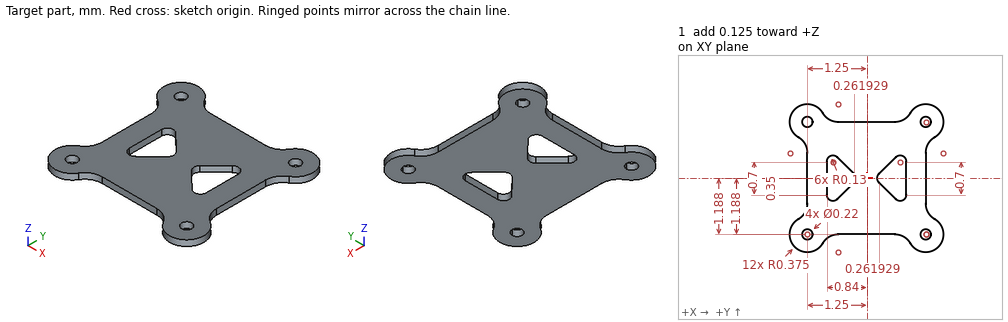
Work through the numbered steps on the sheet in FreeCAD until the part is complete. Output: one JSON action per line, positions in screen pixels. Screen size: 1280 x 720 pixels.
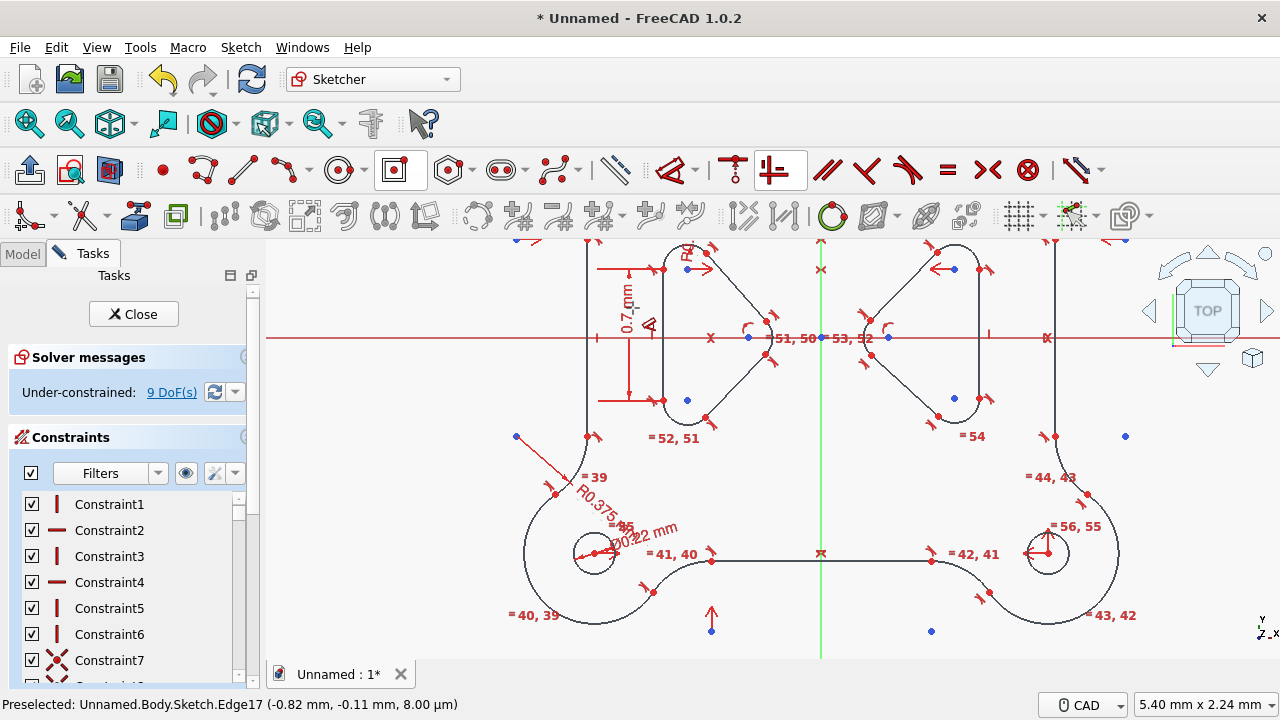
{"action": "left_click", "coordinate": [979, 308]}
{"action": "left_click", "coordinate": [1013, 304]}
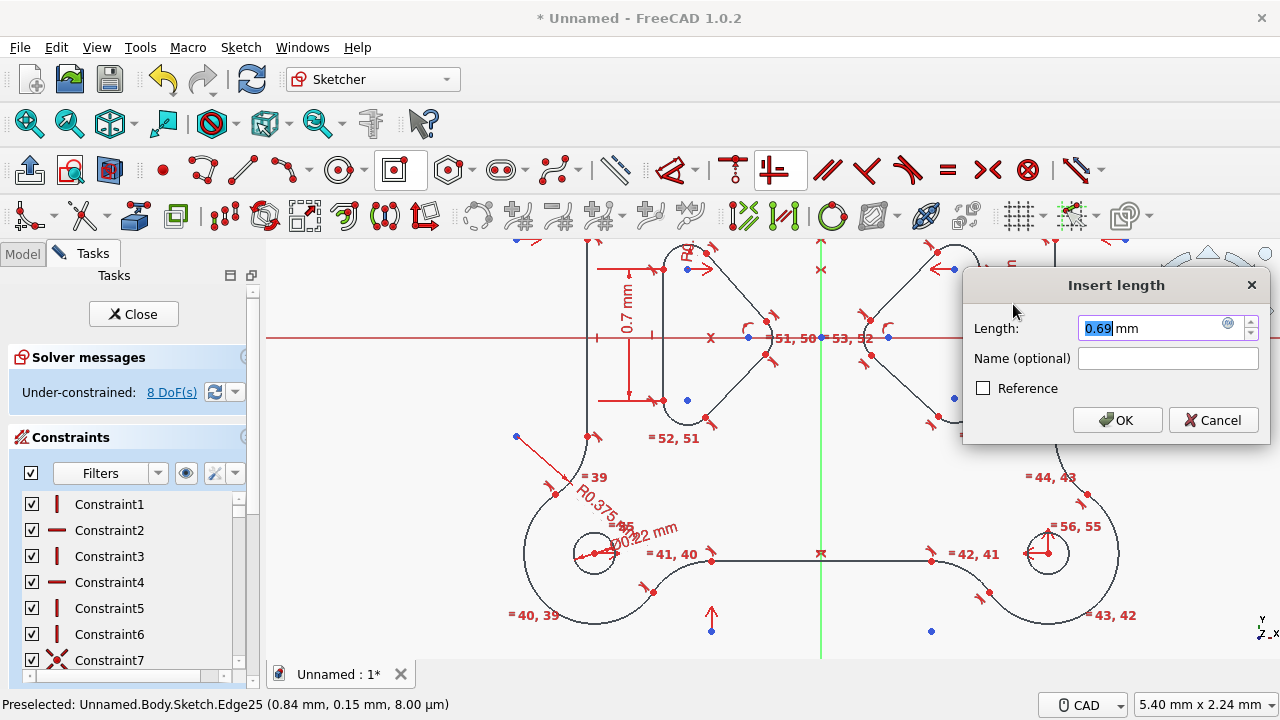
{"action": "type", "text": "0.7"}
{"action": "key", "text": "Return"}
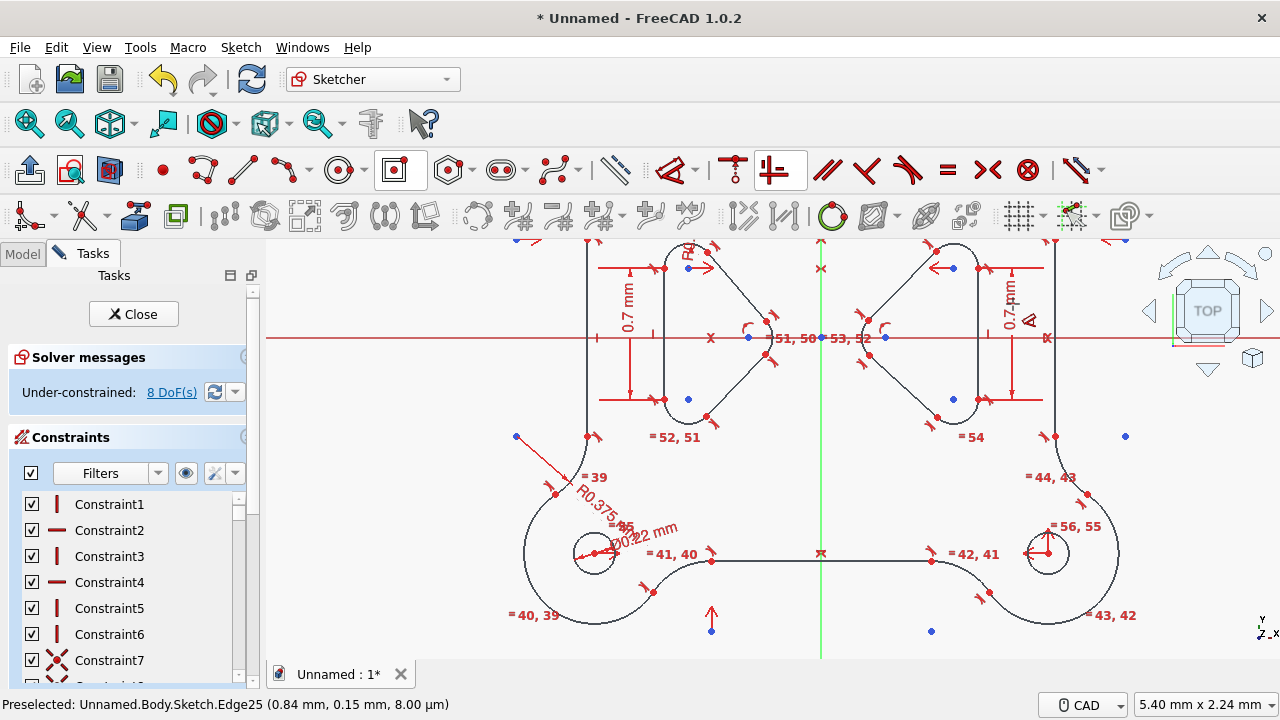
{"action": "left_click", "coordinate": [594, 553]}
{"action": "left_click", "coordinate": [708, 587]}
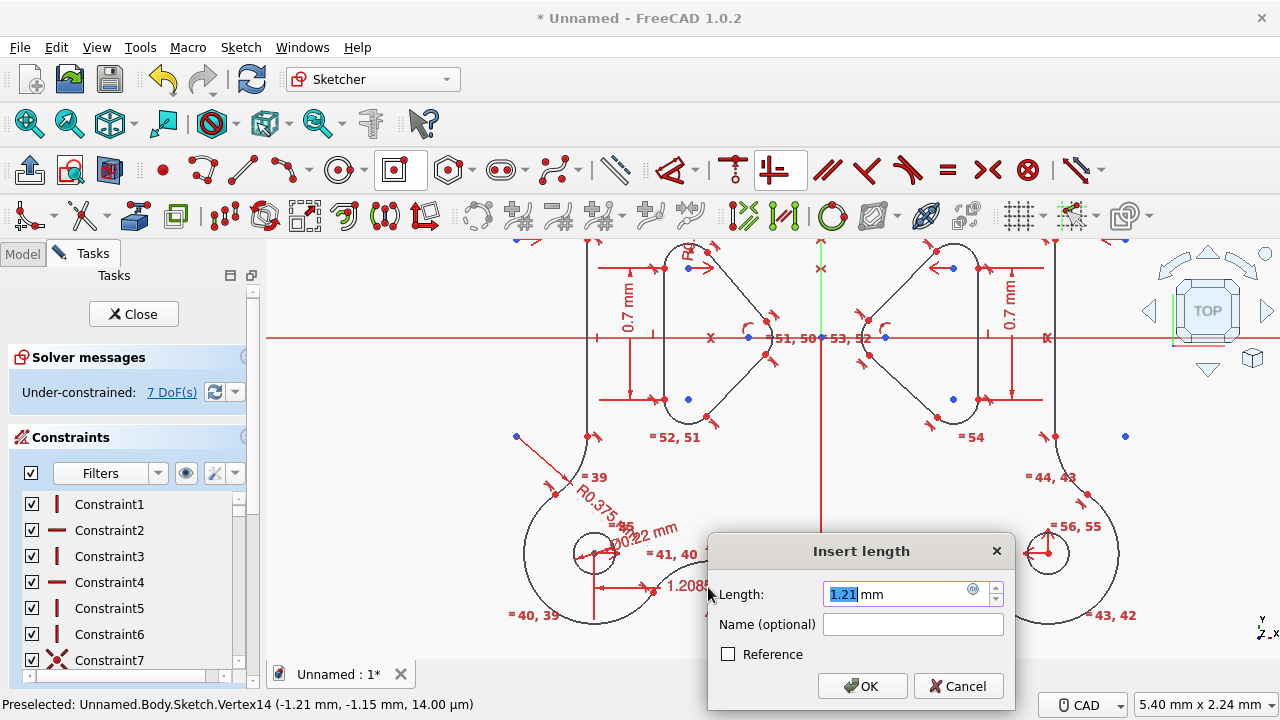
{"action": "type", "text": "1.25"}
{"action": "key", "text": "Return"}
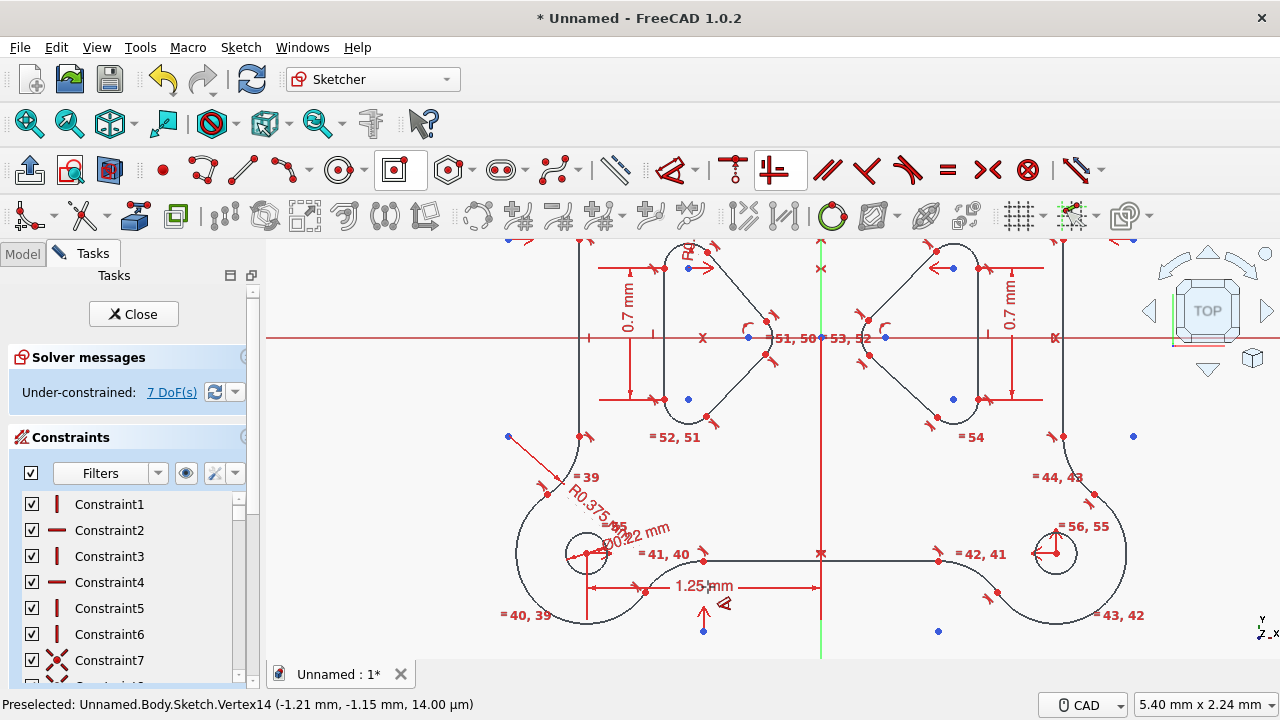
{"action": "scroll", "coordinate": [609, 540], "scroll_direction": "down", "scroll_amount": 4}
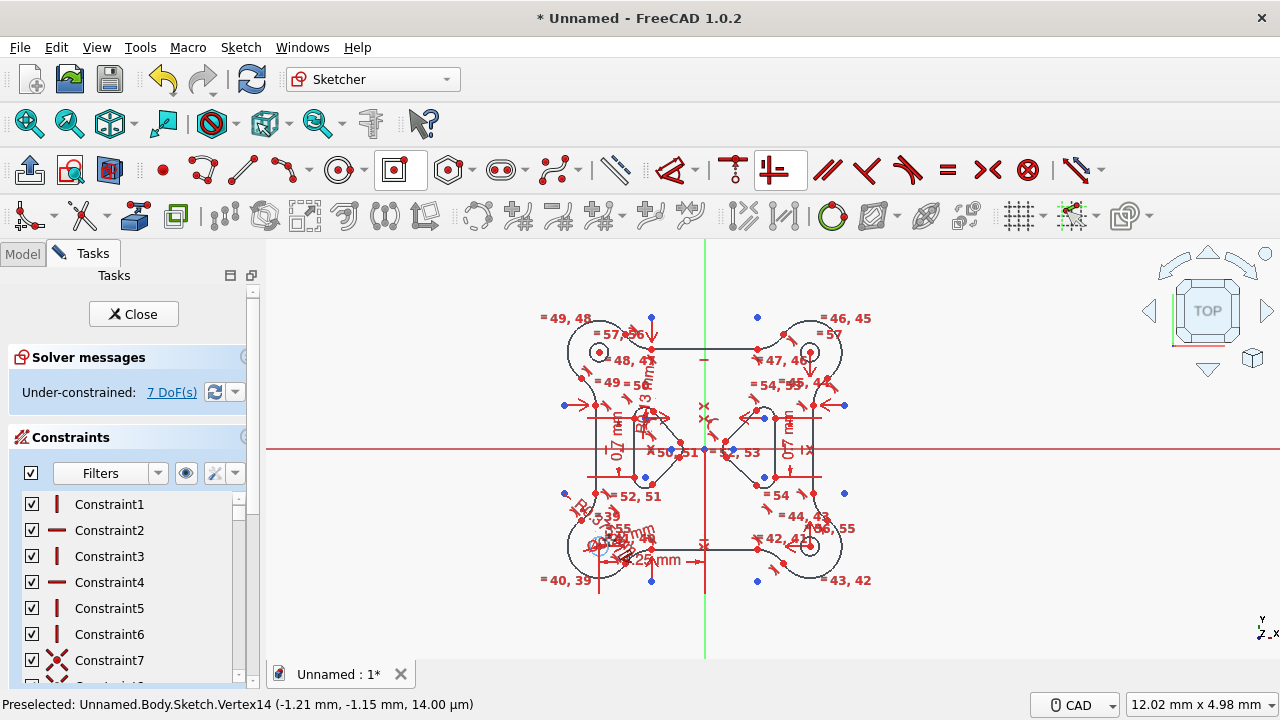
{"action": "left_click", "coordinate": [596, 405]}
{"action": "left_click", "coordinate": [650, 371]}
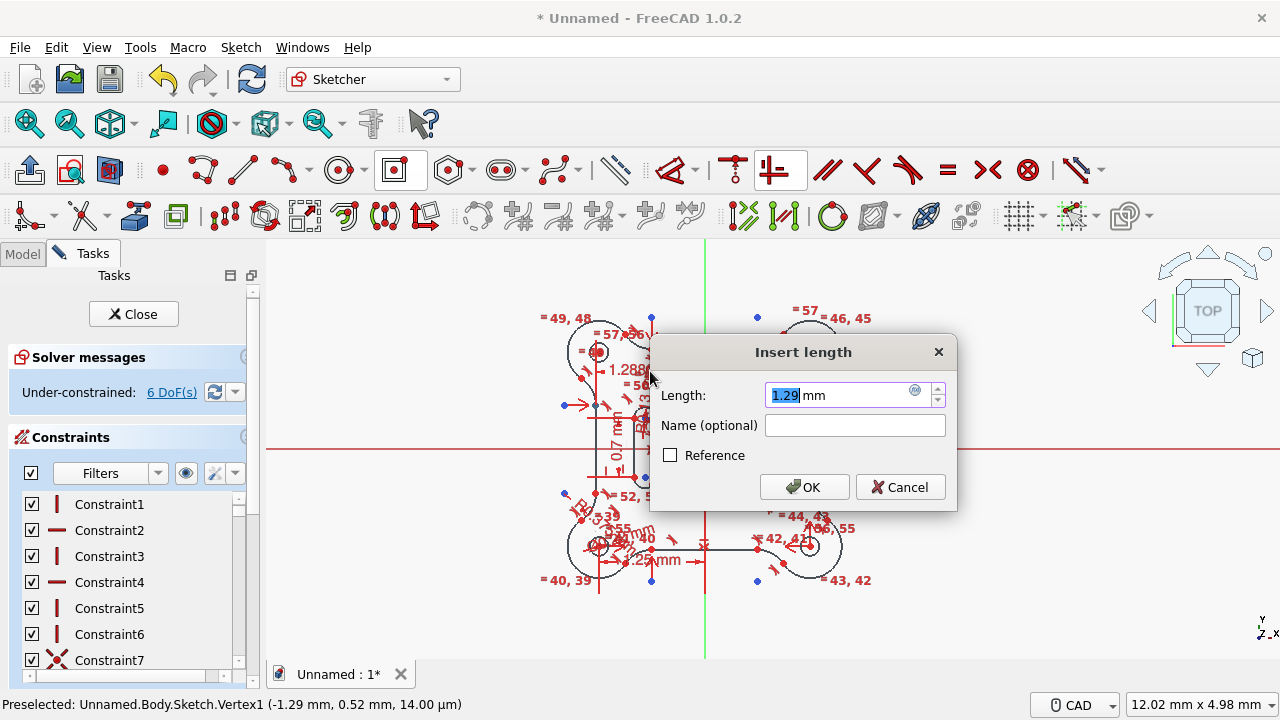
{"action": "type", "text": "1.25"}
{"action": "key", "text": "Return"}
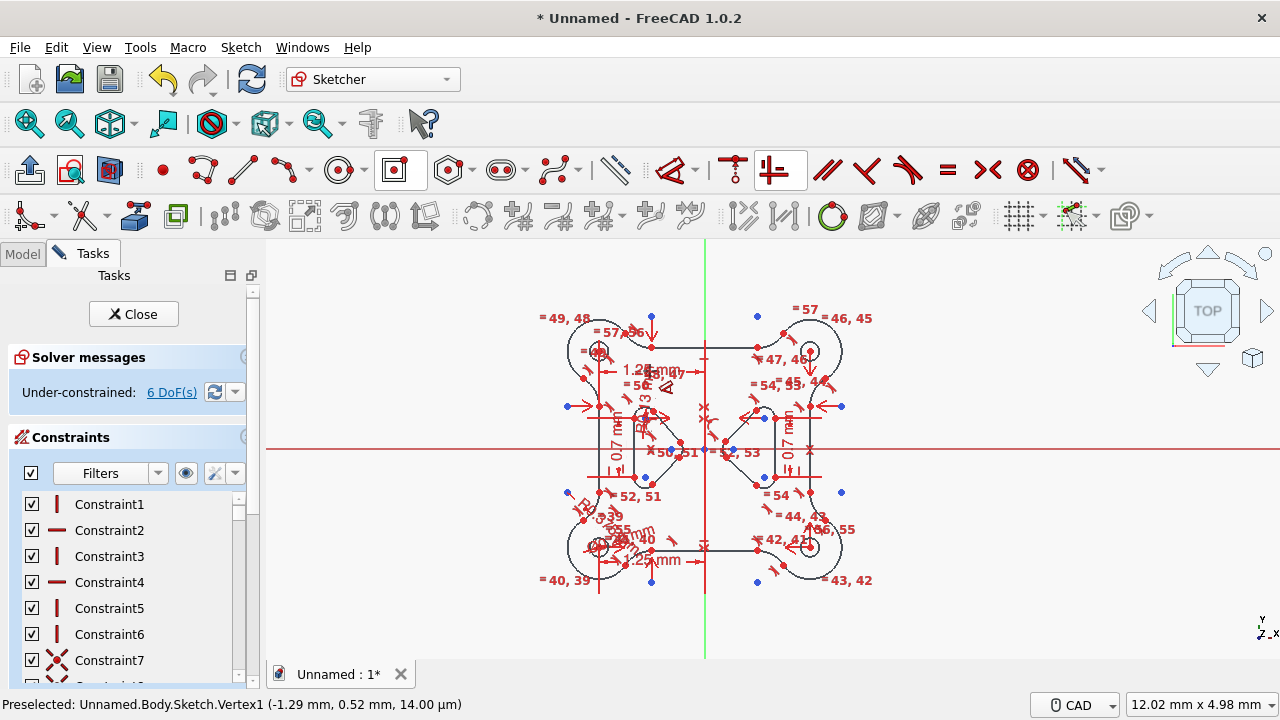
{"action": "left_click", "coordinate": [634, 477]}
{"action": "left_click", "coordinate": [686, 511]}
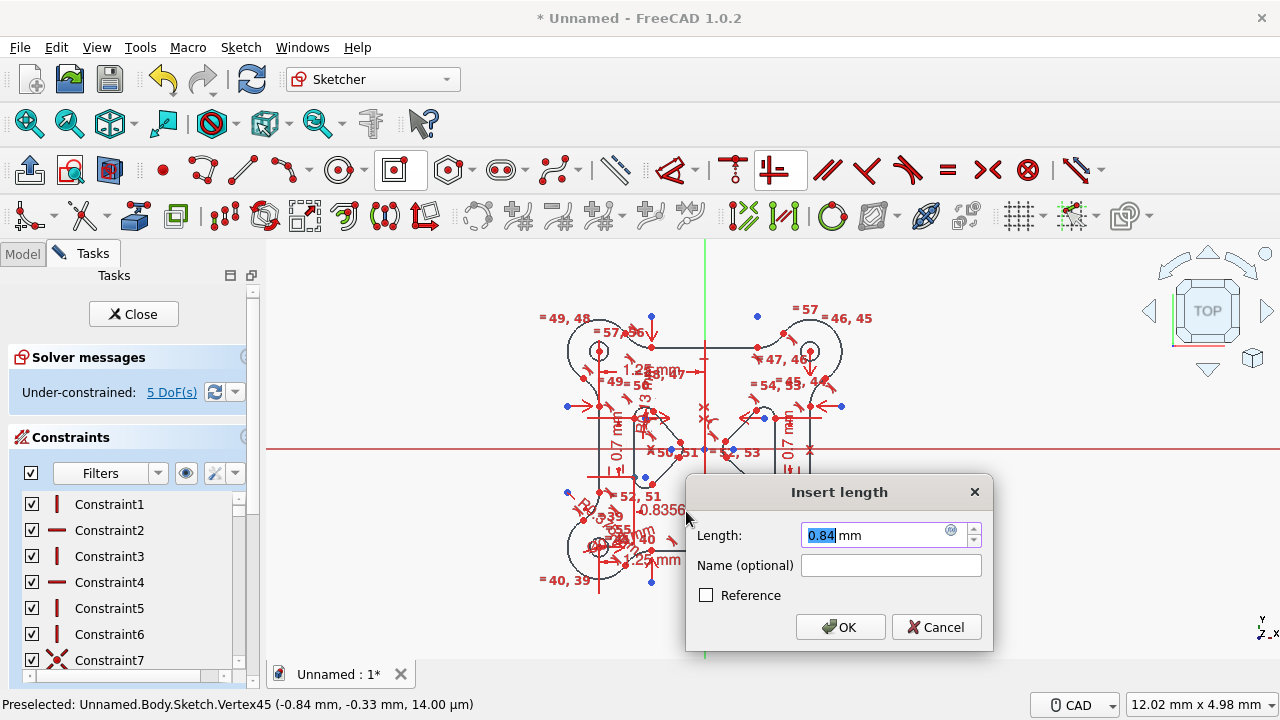
{"action": "type", "text": "0.84"}
{"action": "key", "text": "Return"}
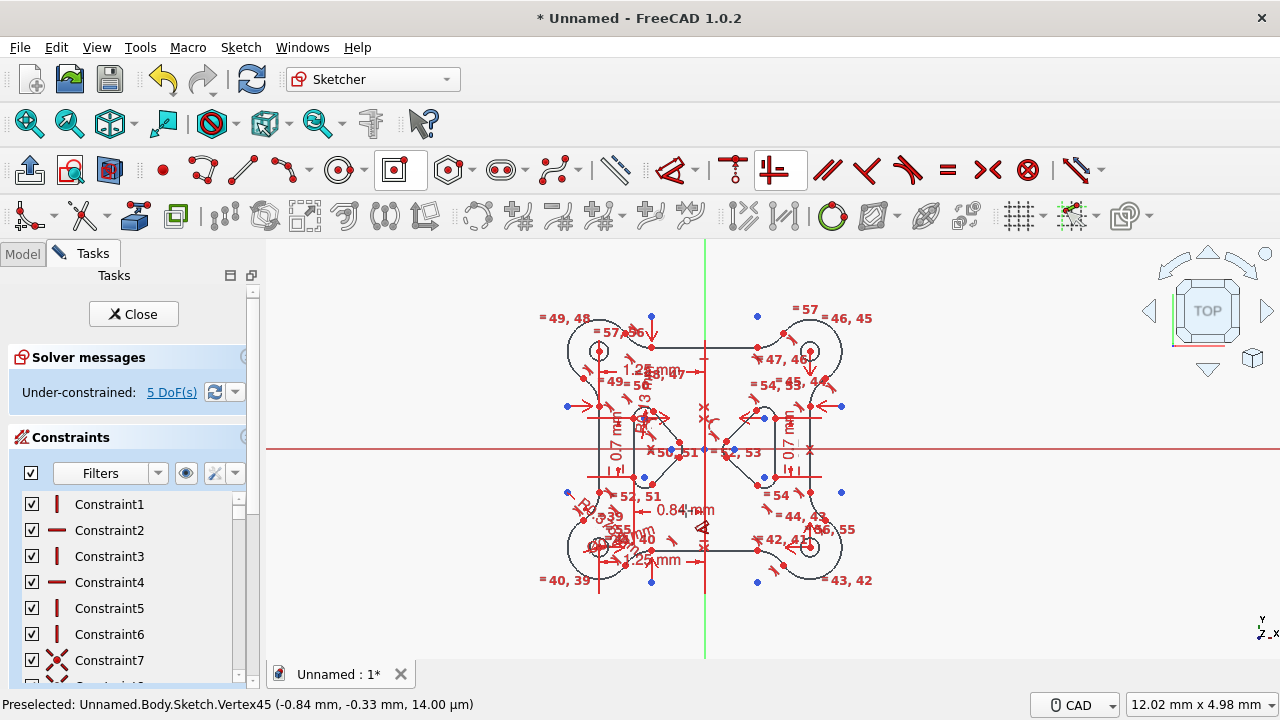
{"action": "scroll", "coordinate": [634, 477], "scroll_direction": "up", "scroll_amount": 2}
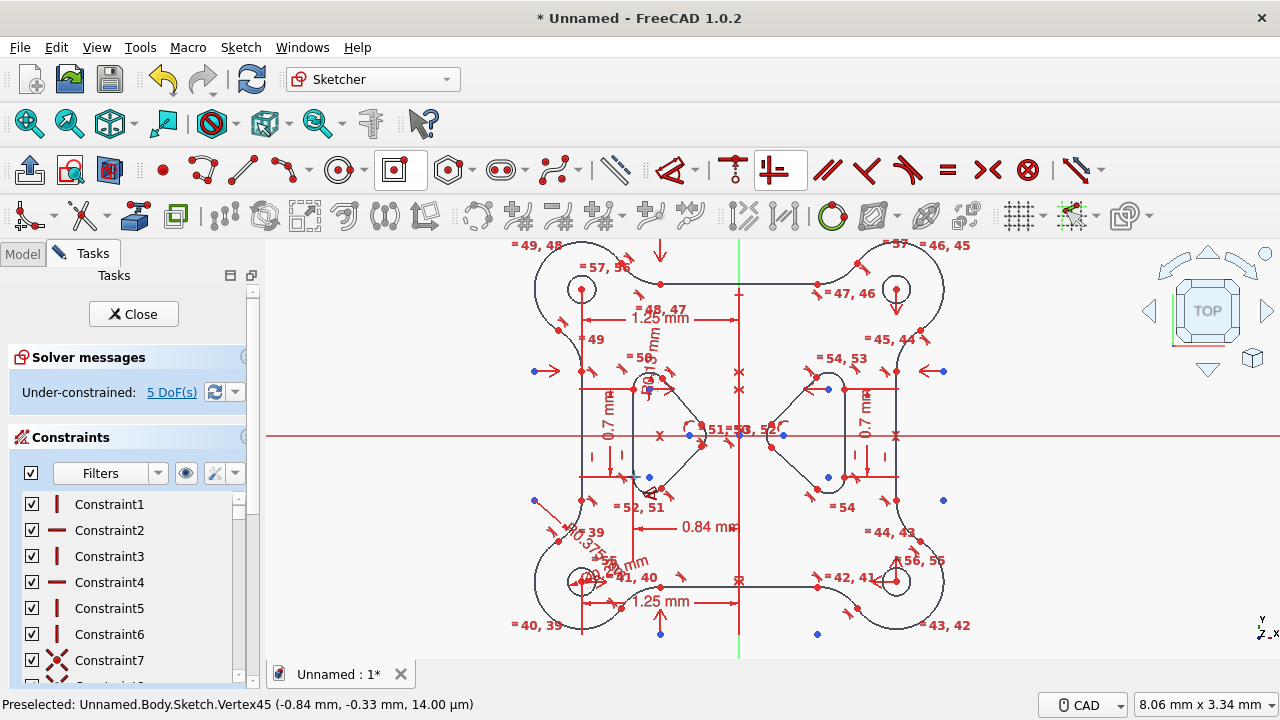
{"action": "left_click", "coordinate": [633, 477]}
{"action": "left_click", "coordinate": [599, 456]}